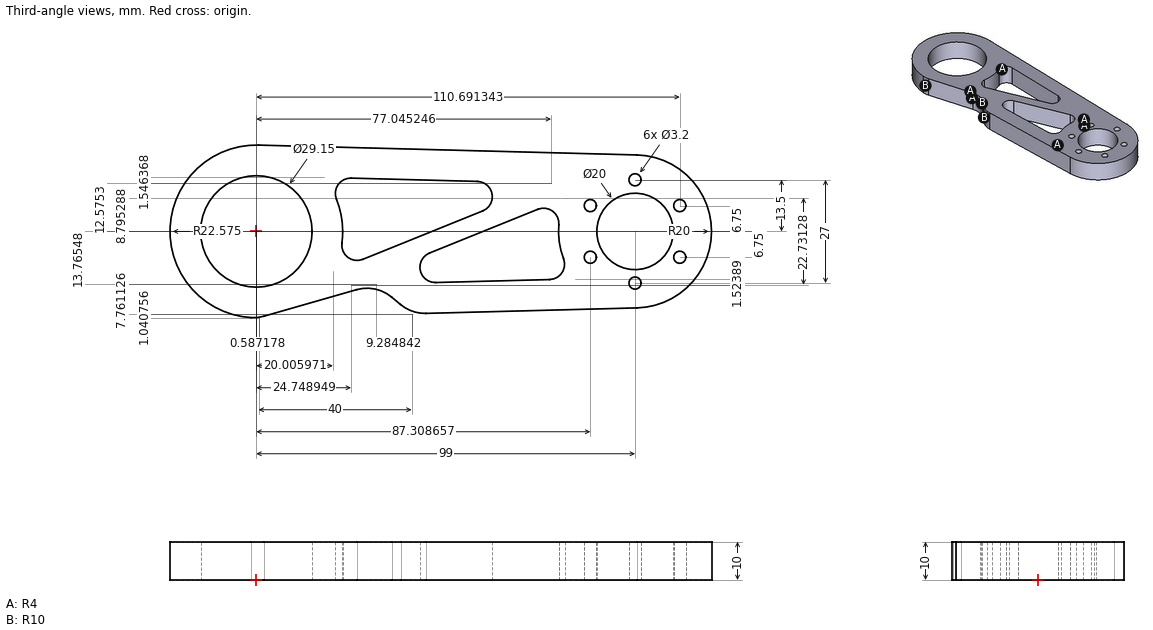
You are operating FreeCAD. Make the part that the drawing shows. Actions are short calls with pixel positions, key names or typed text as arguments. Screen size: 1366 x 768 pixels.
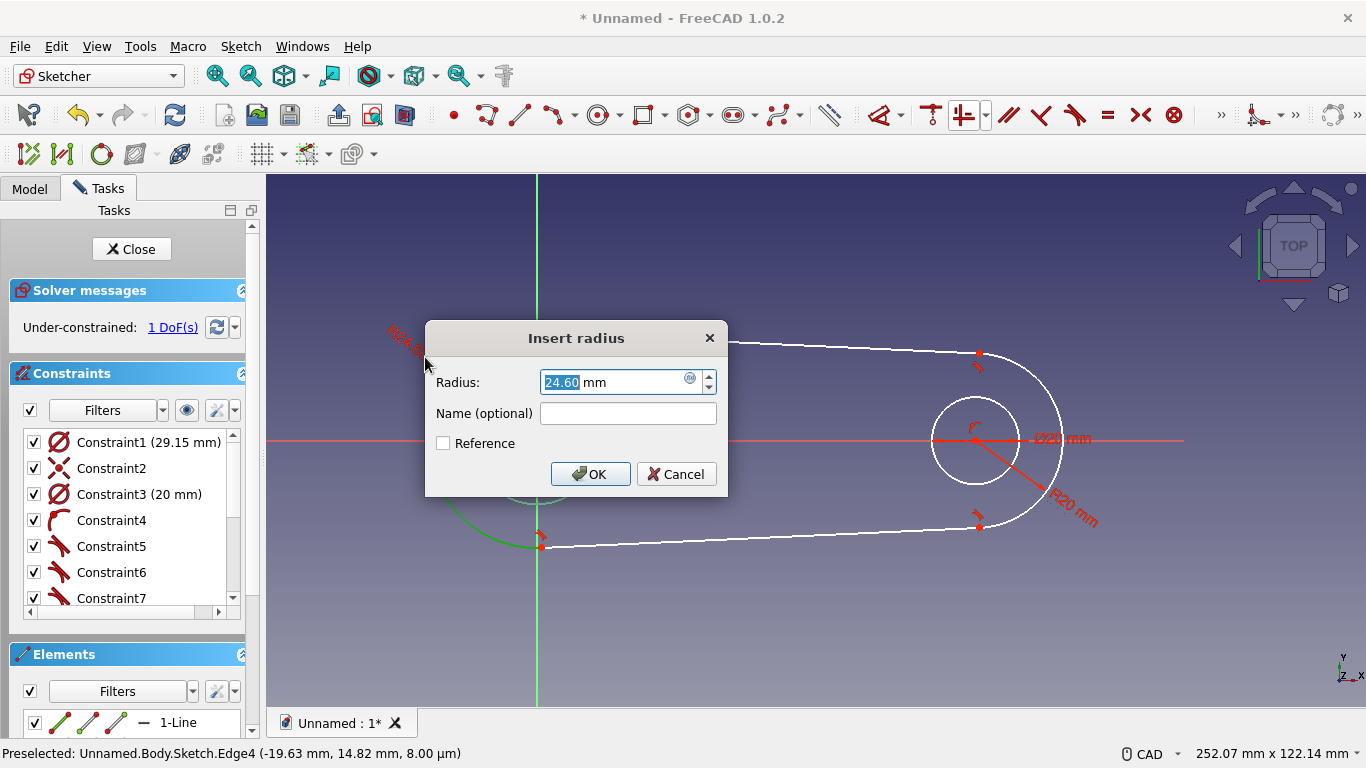
text(22.575)
key(Return)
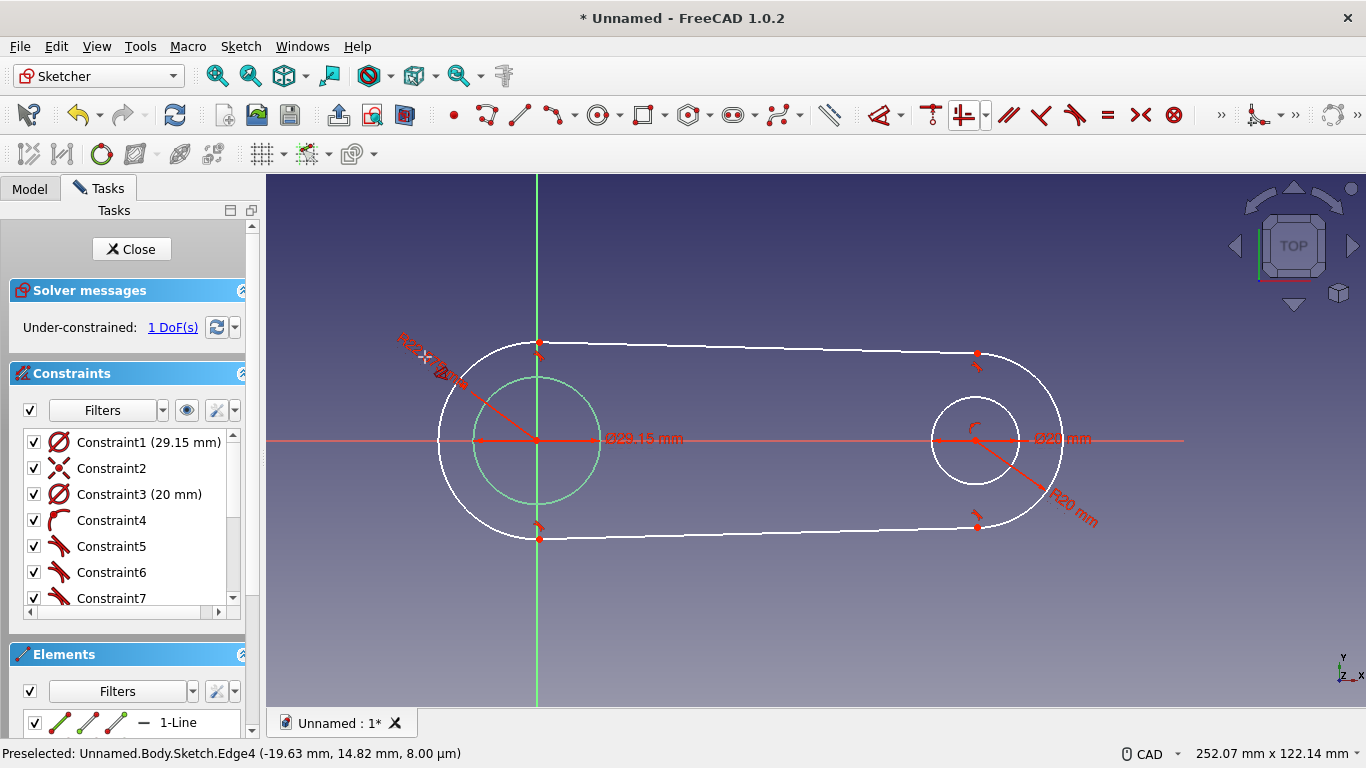
click(976, 441)
click(756, 475)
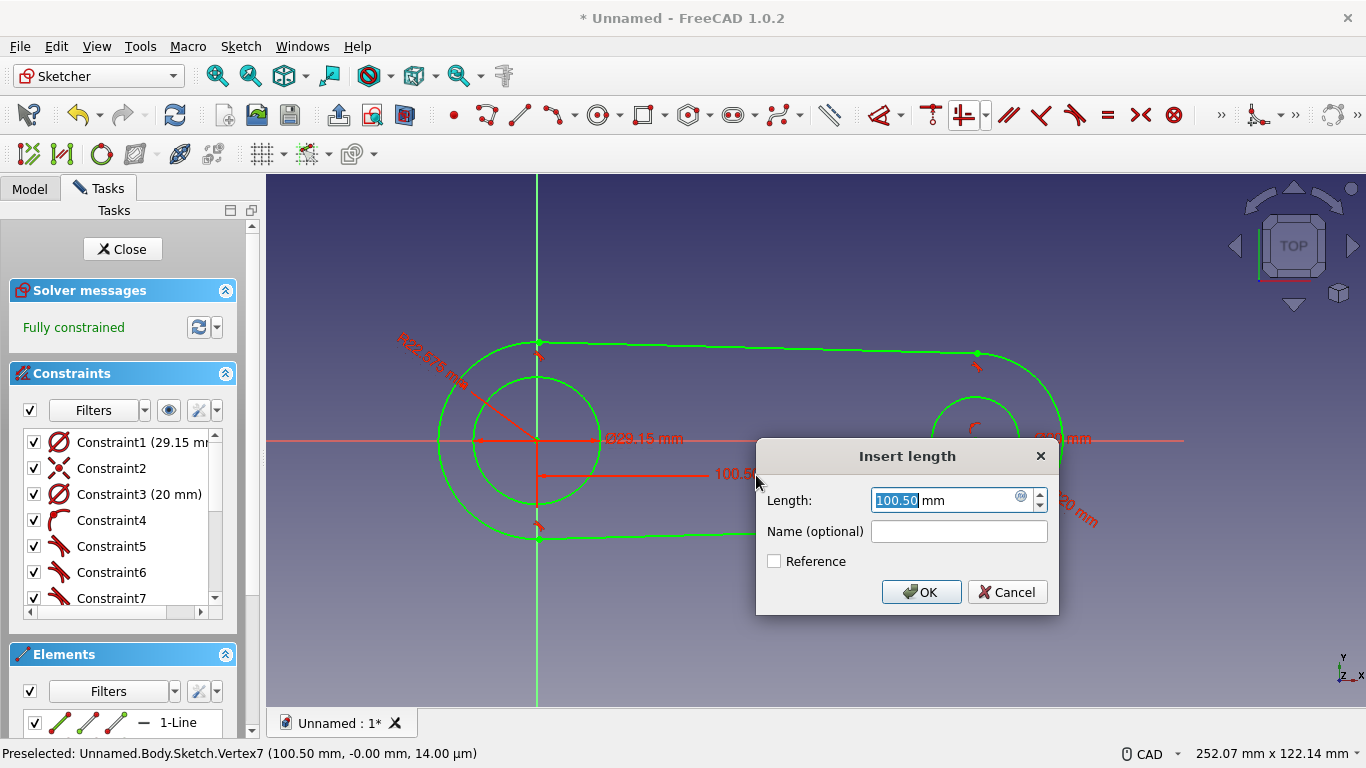
text(99)
key(Return)
key(Escape)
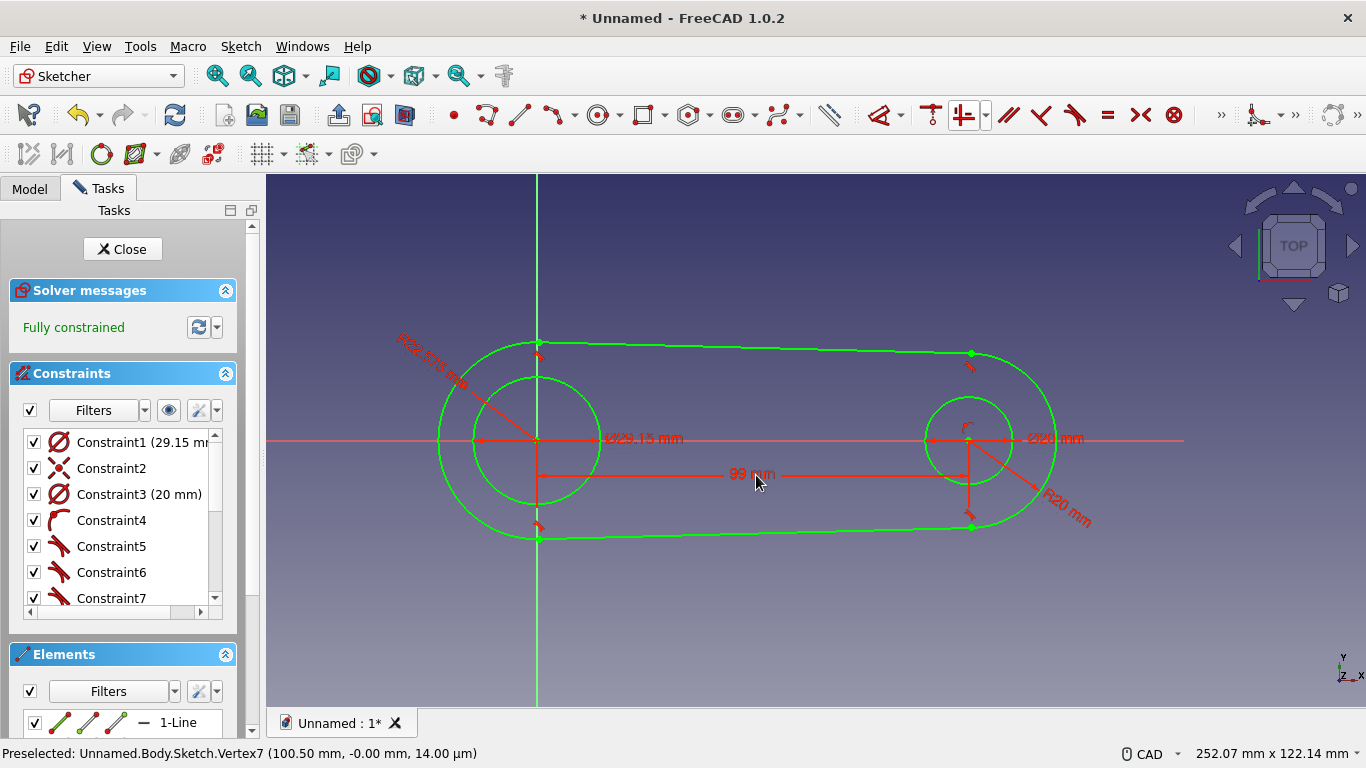
click(123, 249)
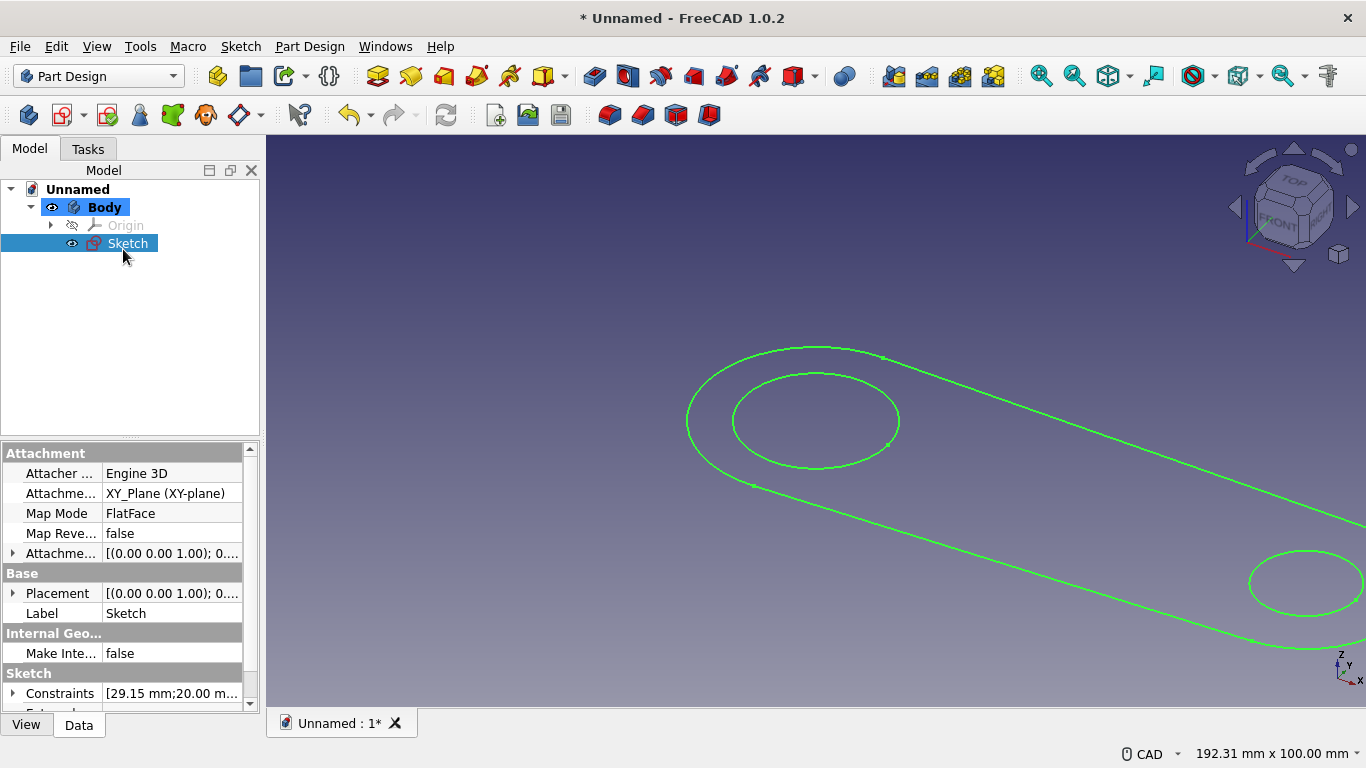
click(378, 76)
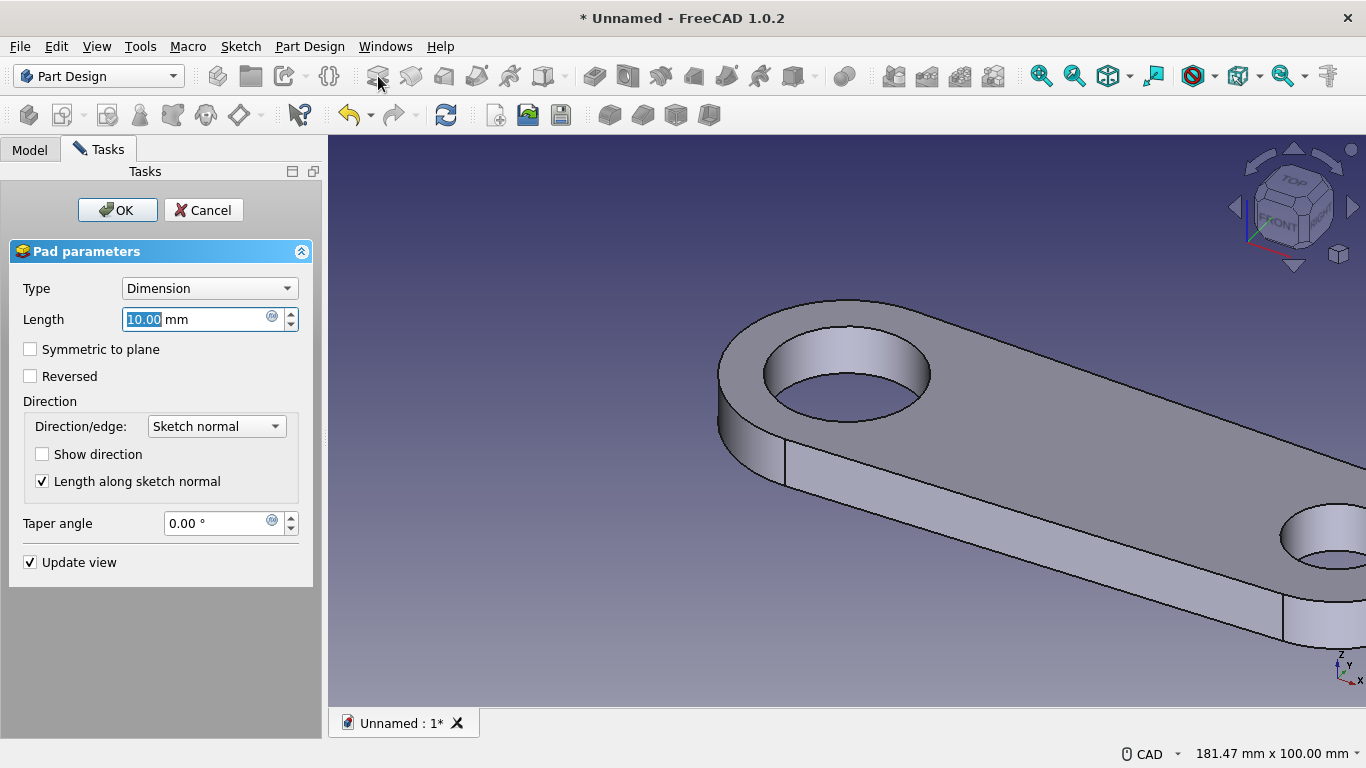
text(10)
key(Tab)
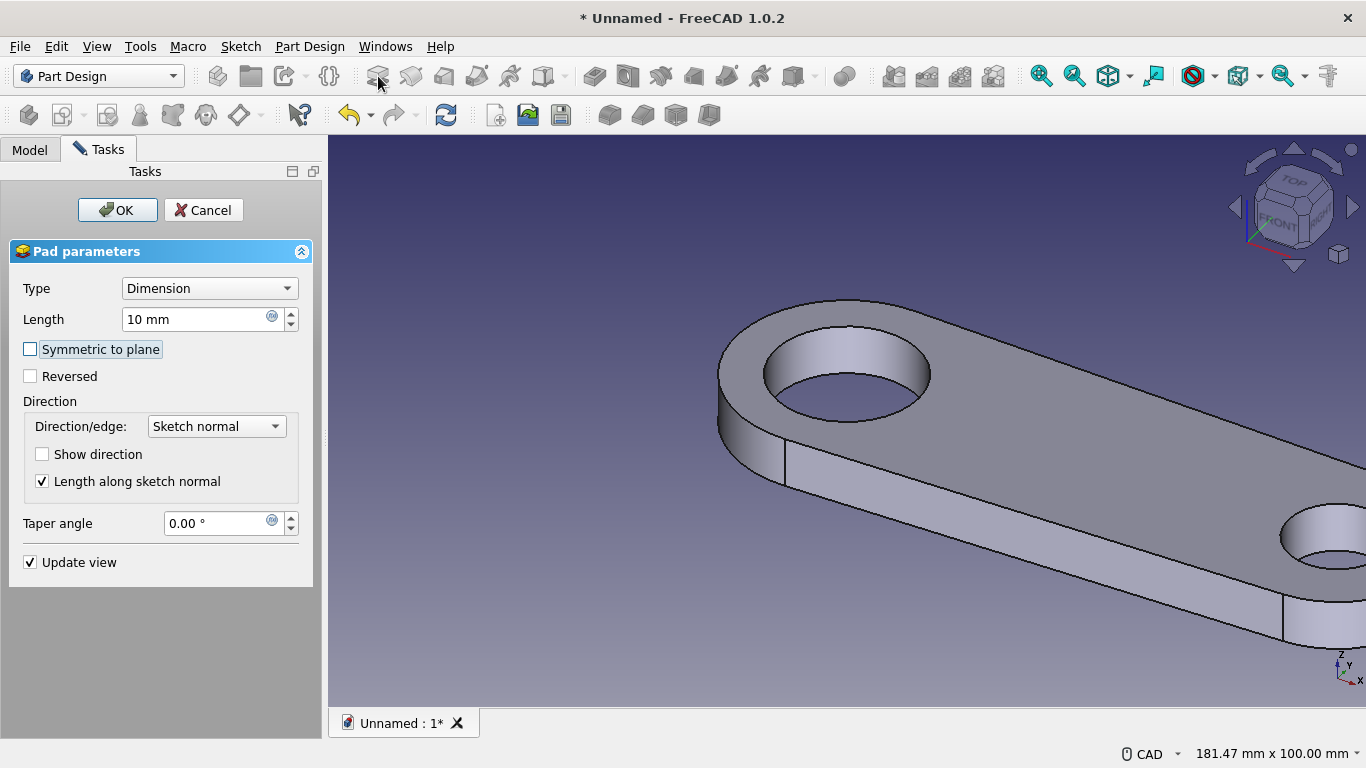
click(118, 210)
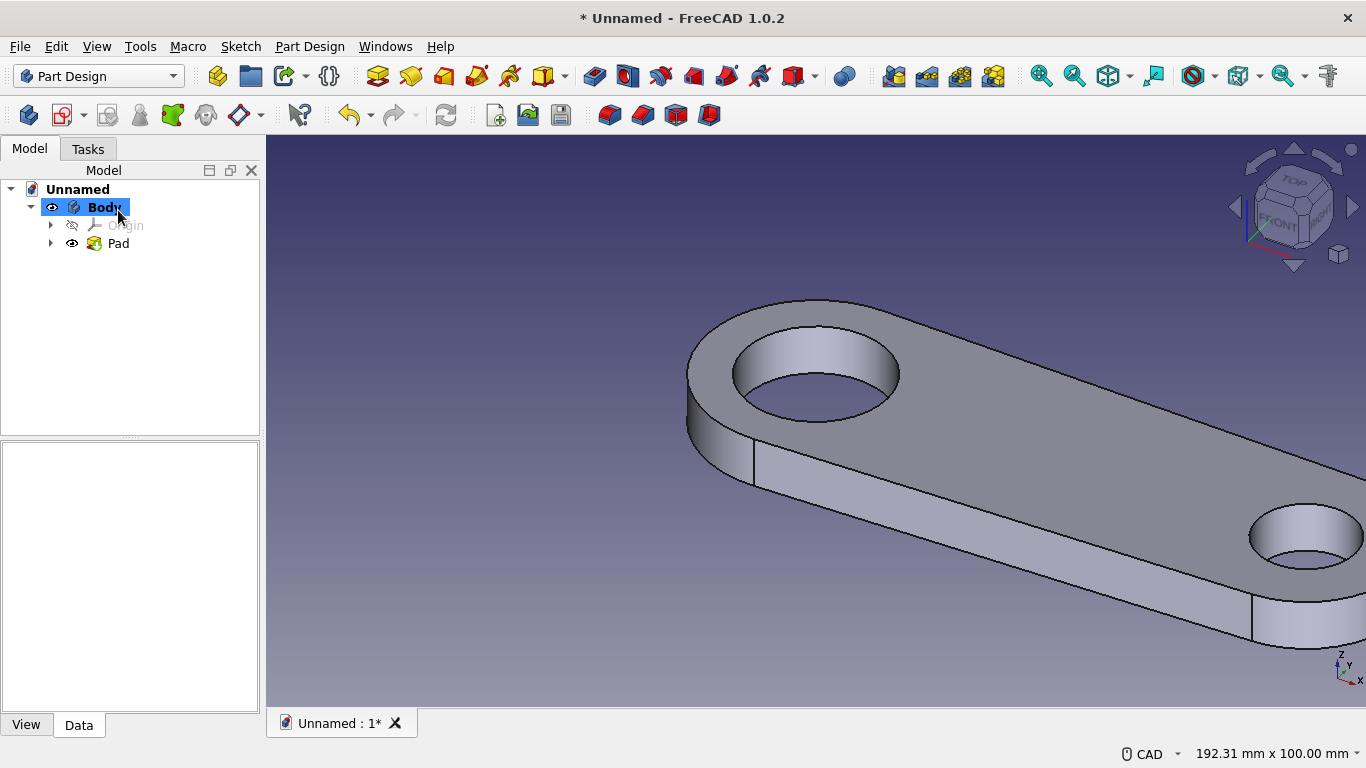
key(v)
key(f)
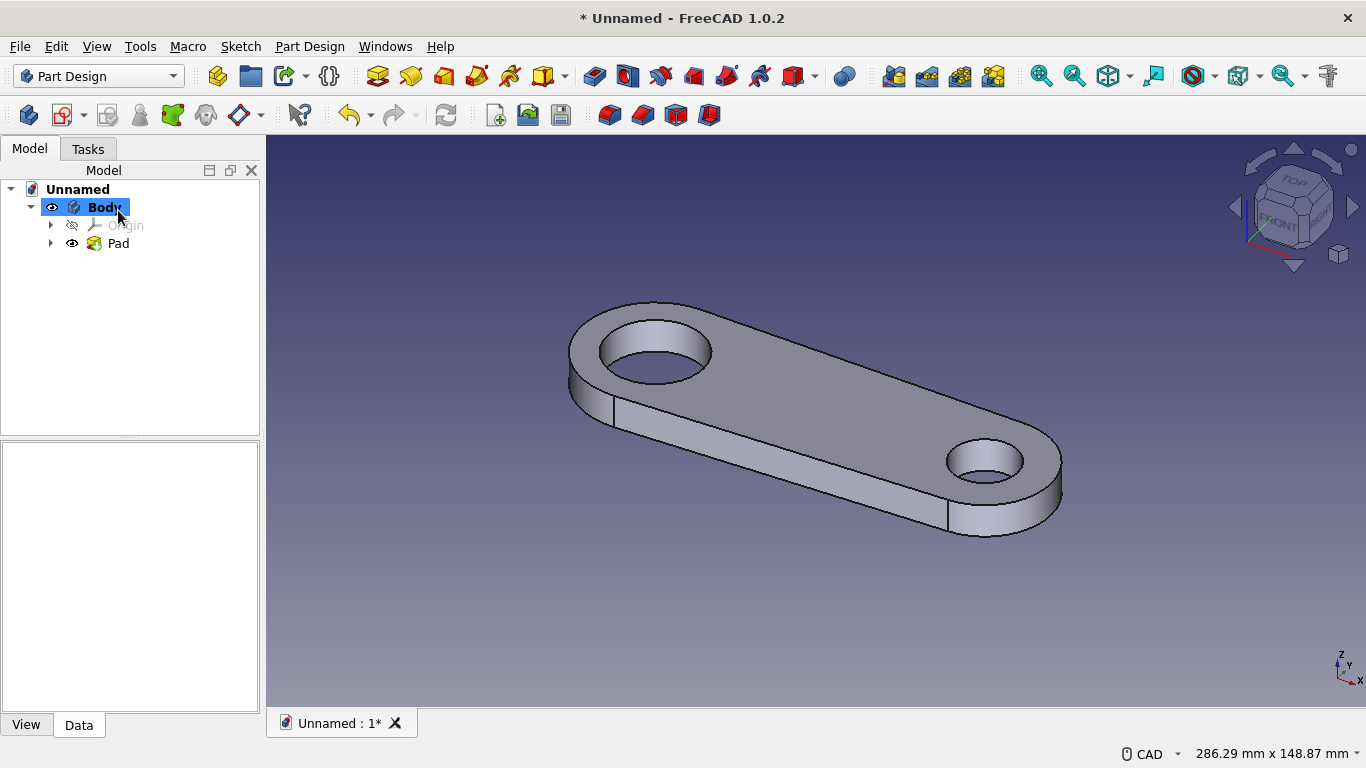
key(5)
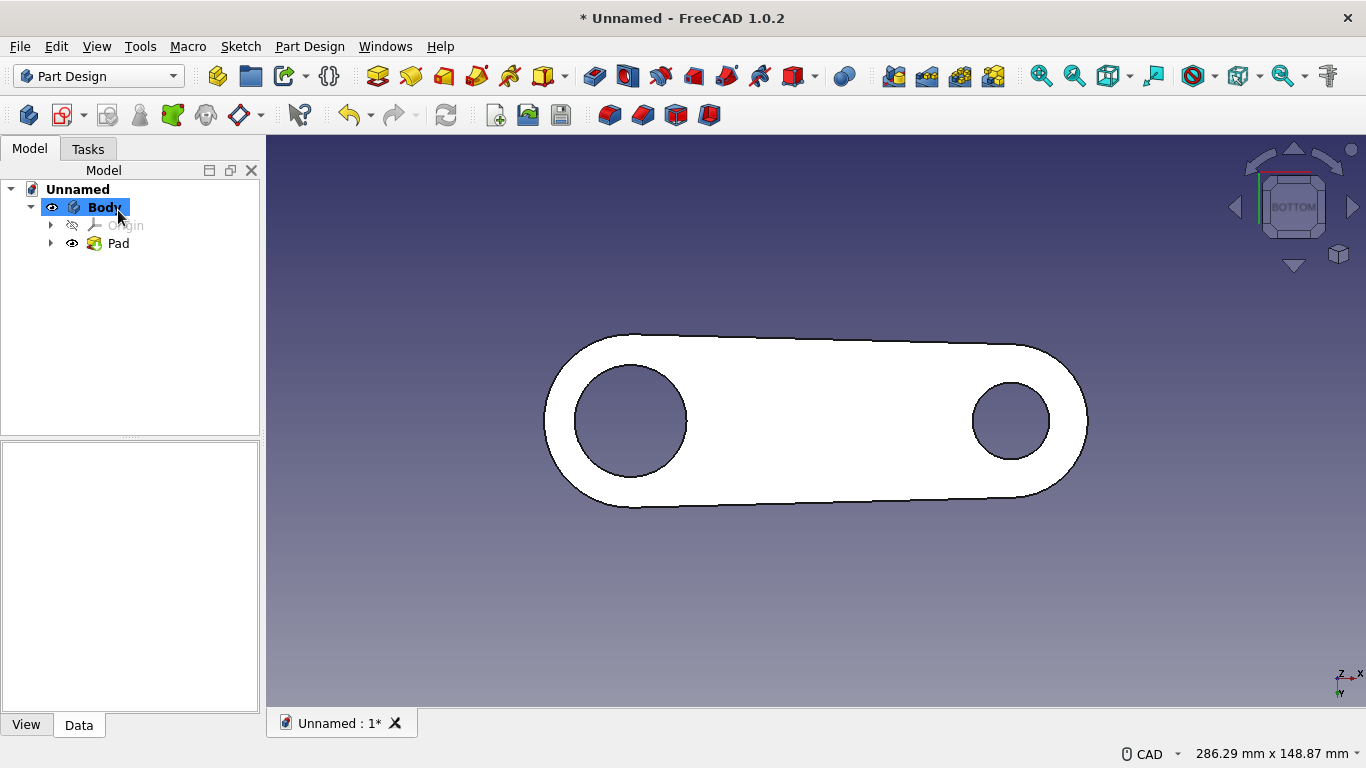
click(816, 420)